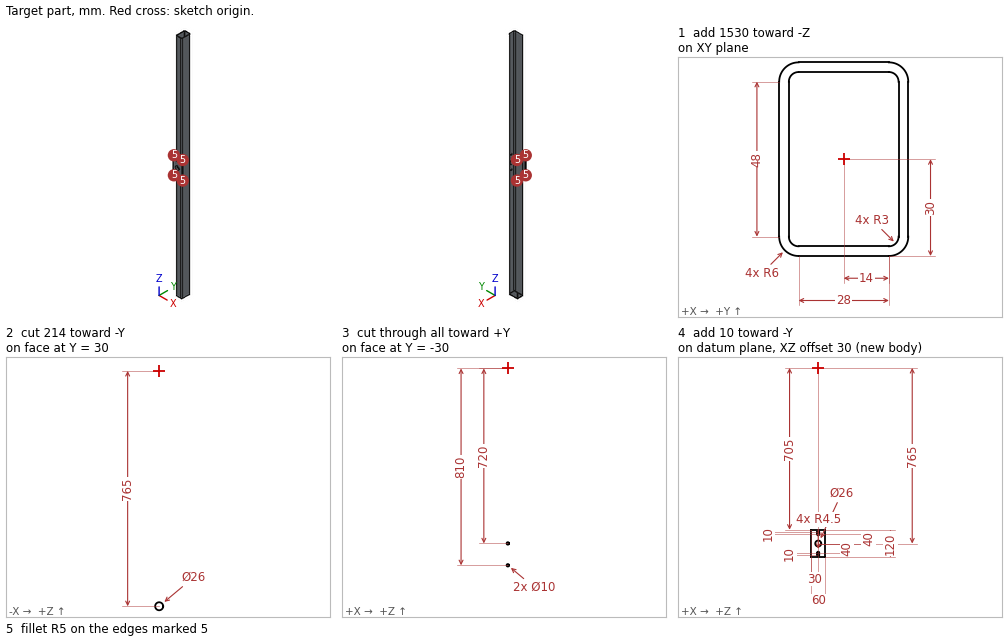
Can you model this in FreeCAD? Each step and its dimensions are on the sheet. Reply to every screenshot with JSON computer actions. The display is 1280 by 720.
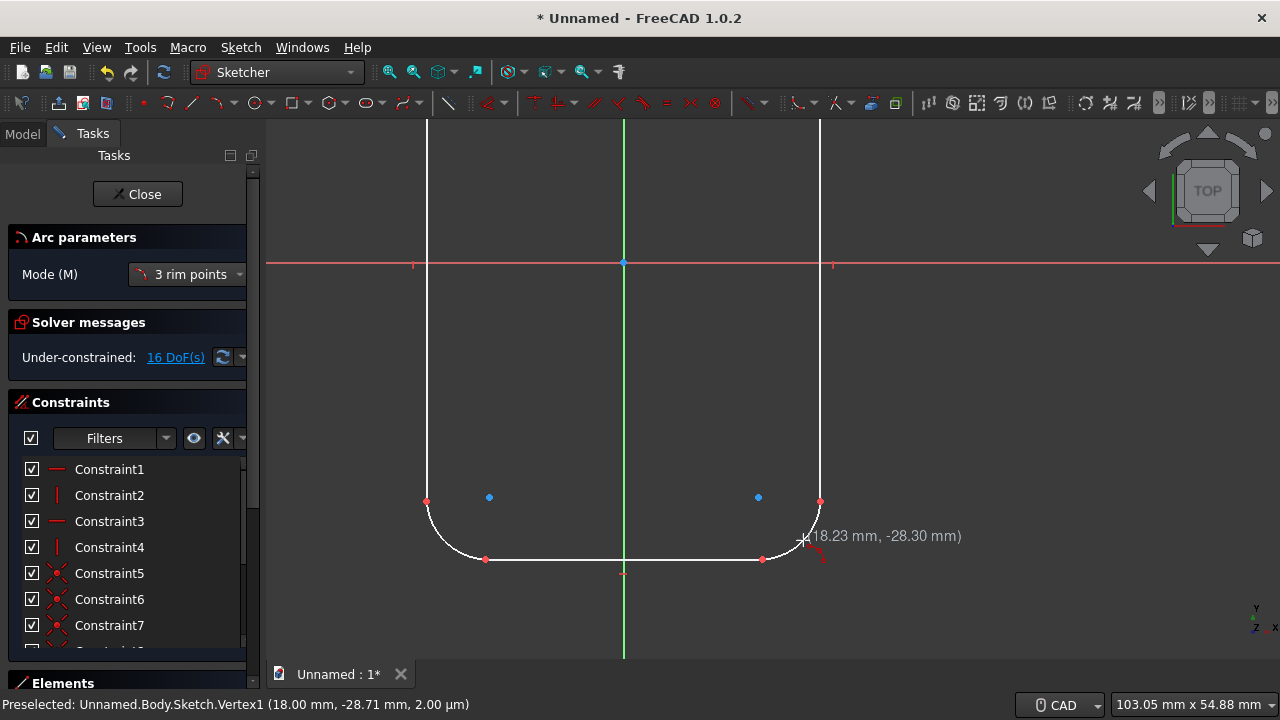
{"action": "left_click", "coordinate": [192, 104]}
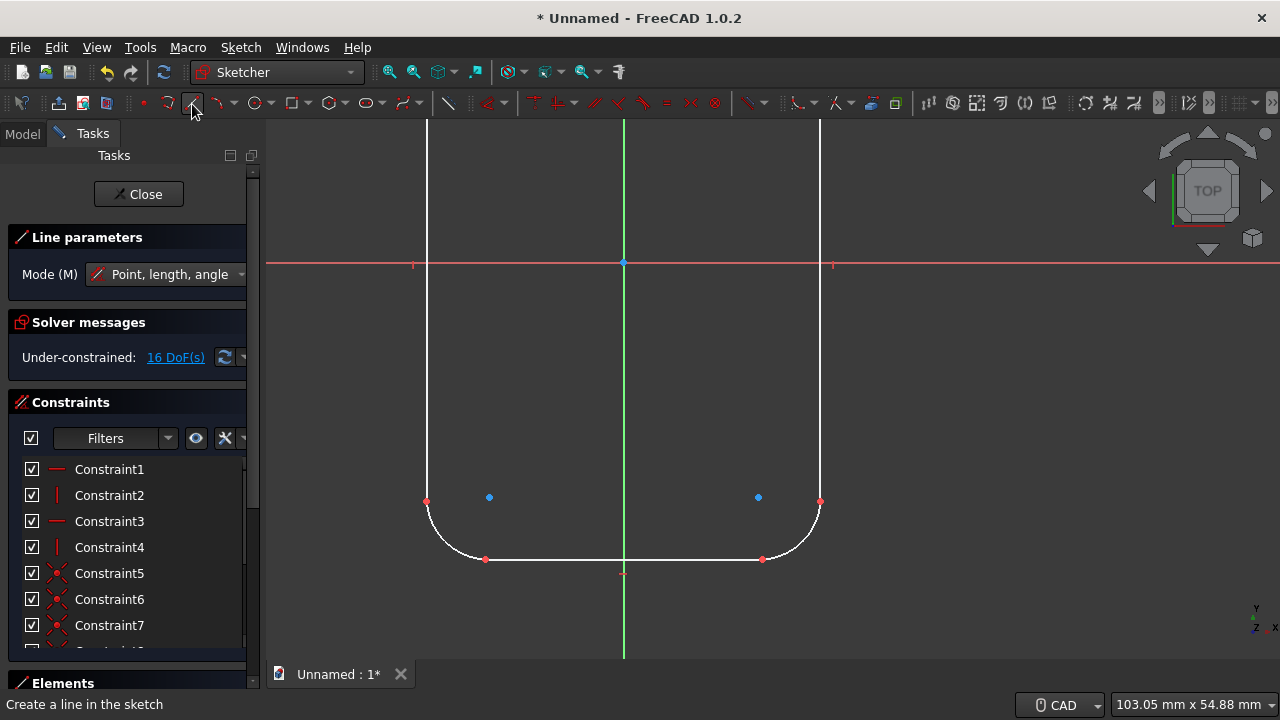
{"action": "left_click", "coordinate": [486, 528]}
{"action": "left_click", "coordinate": [761, 528]}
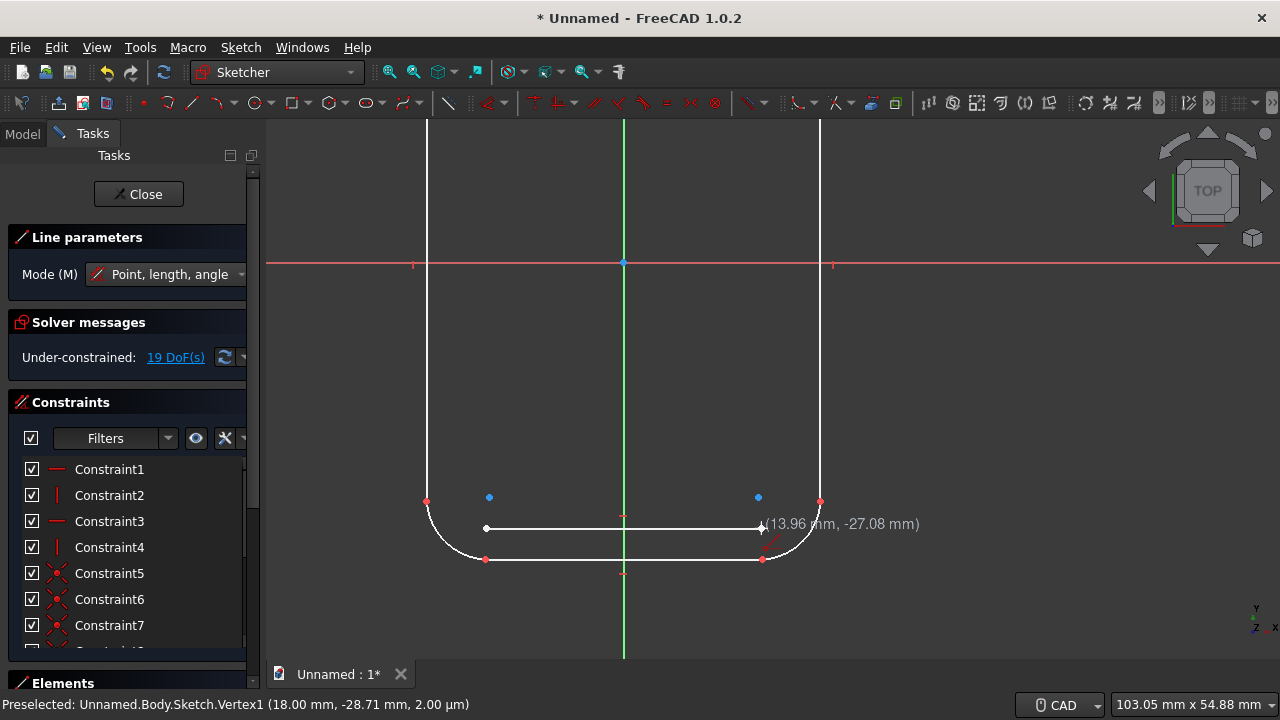
{"action": "left_click", "coordinate": [791, 499]}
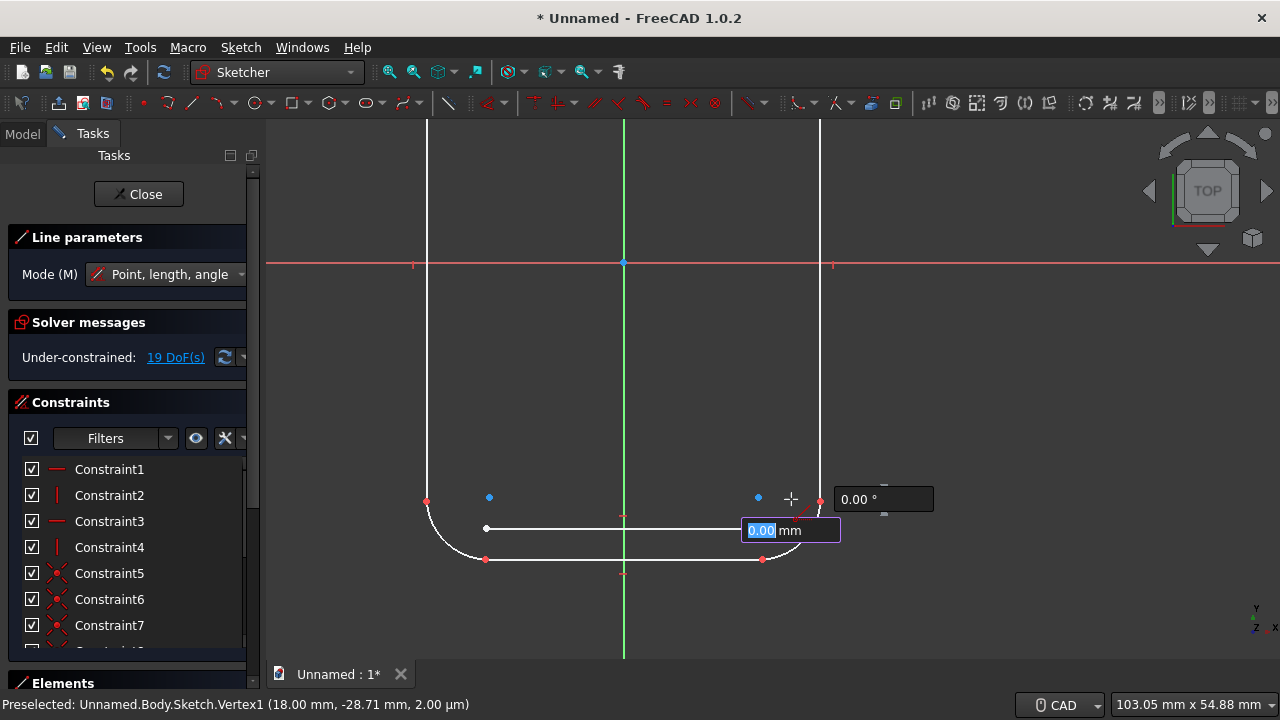
{"action": "scroll", "coordinate": [803, 543], "scroll_direction": "down", "scroll_amount": 3}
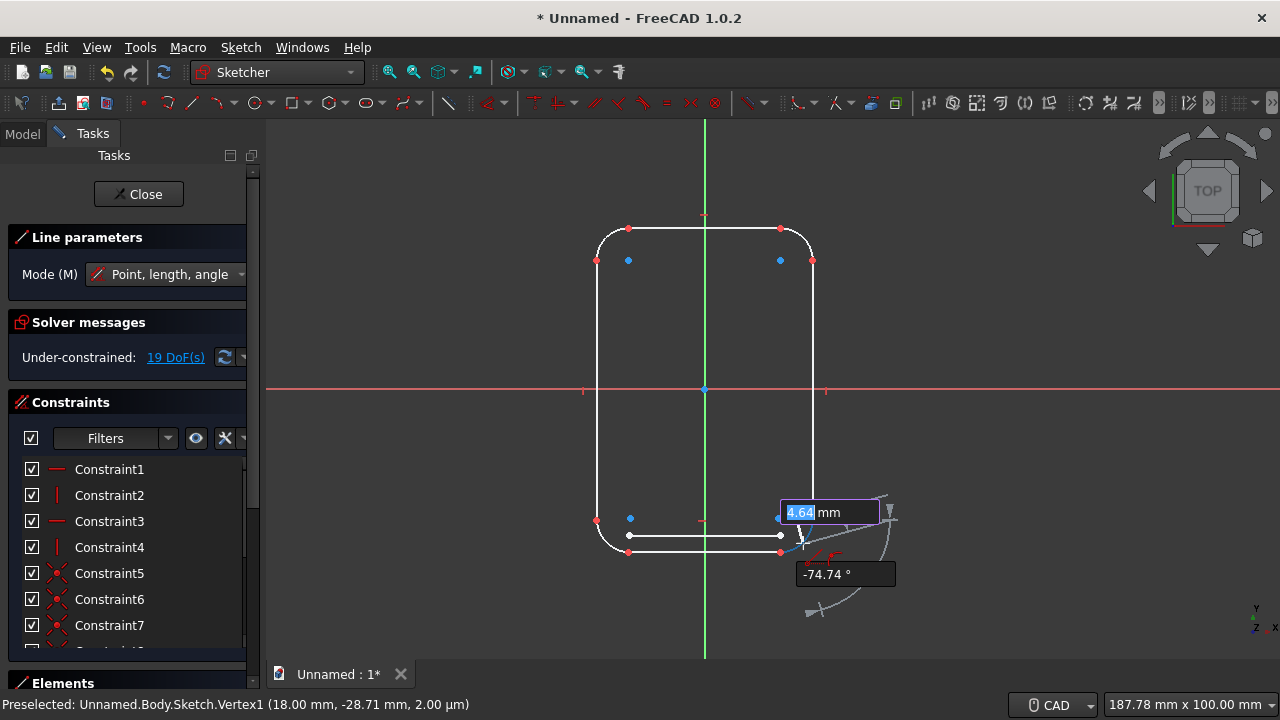
{"action": "left_click", "coordinate": [797, 260]}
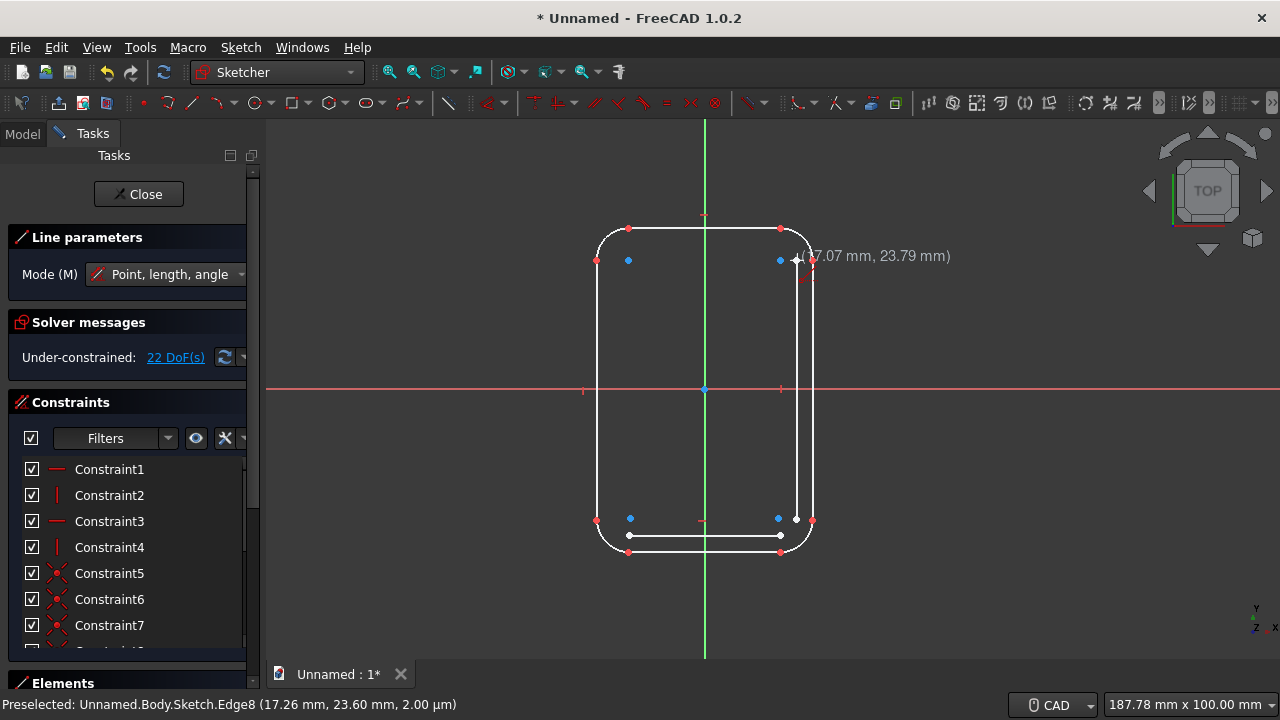
{"action": "left_click", "coordinate": [780, 244]}
{"action": "left_click", "coordinate": [629, 244]}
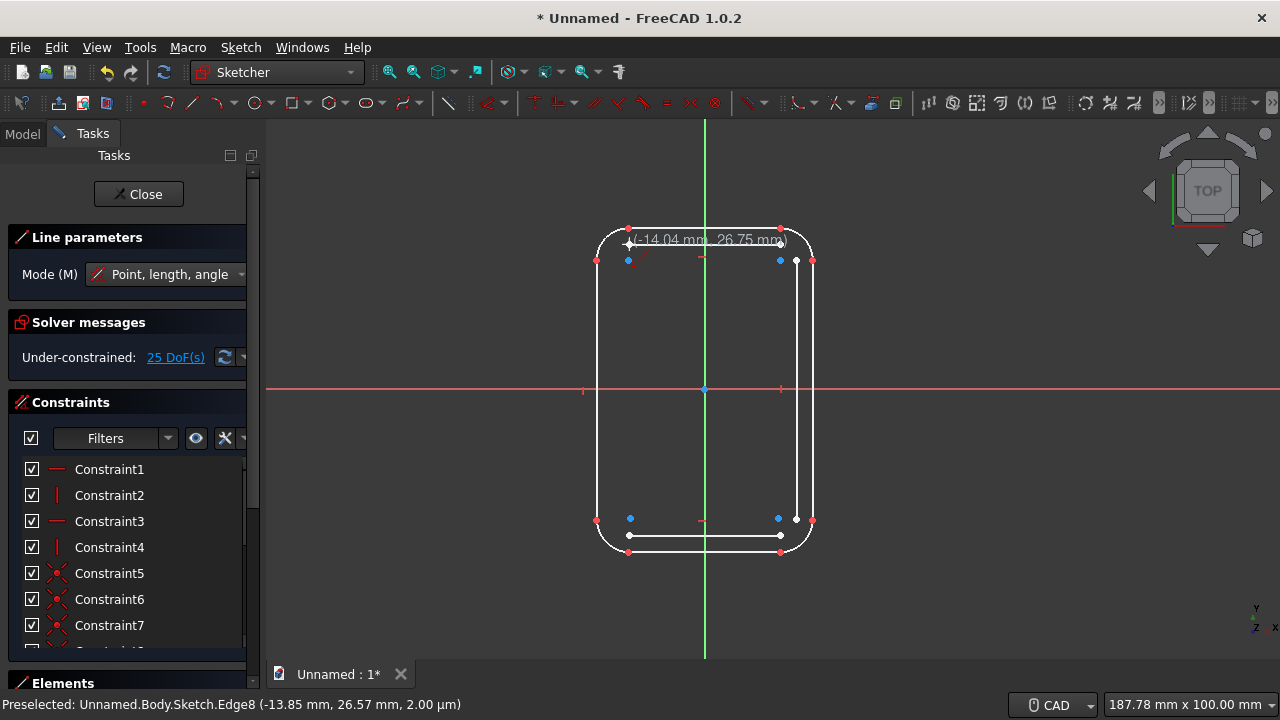
{"action": "left_click", "coordinate": [613, 260]}
{"action": "left_click", "coordinate": [613, 519]}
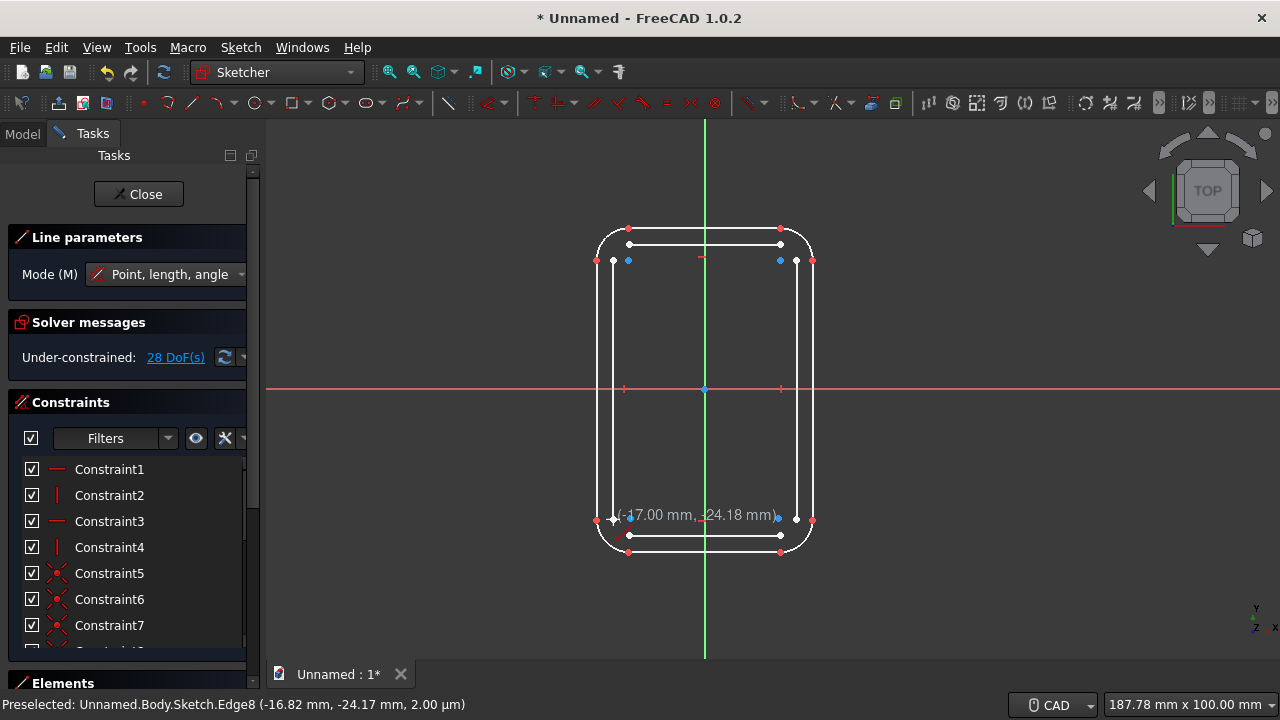
{"action": "left_click", "coordinate": [218, 104]}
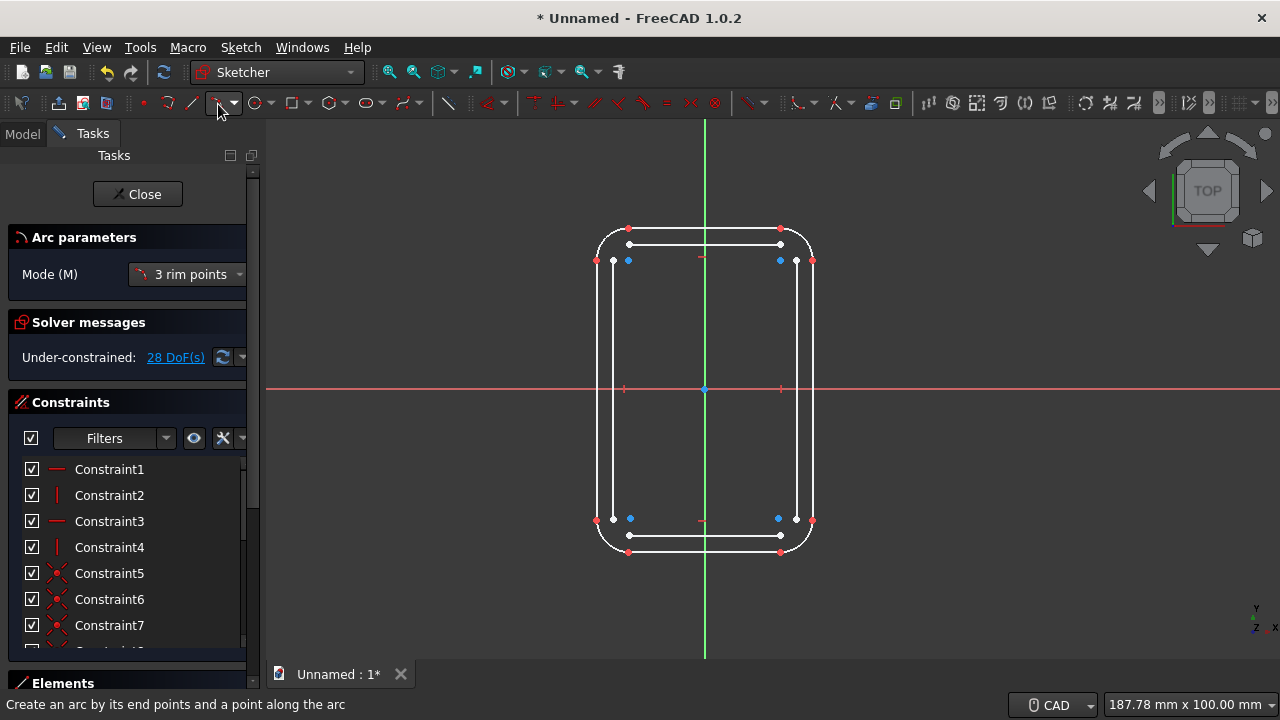
{"action": "left_click", "coordinate": [780, 536]}
{"action": "left_click", "coordinate": [797, 520]}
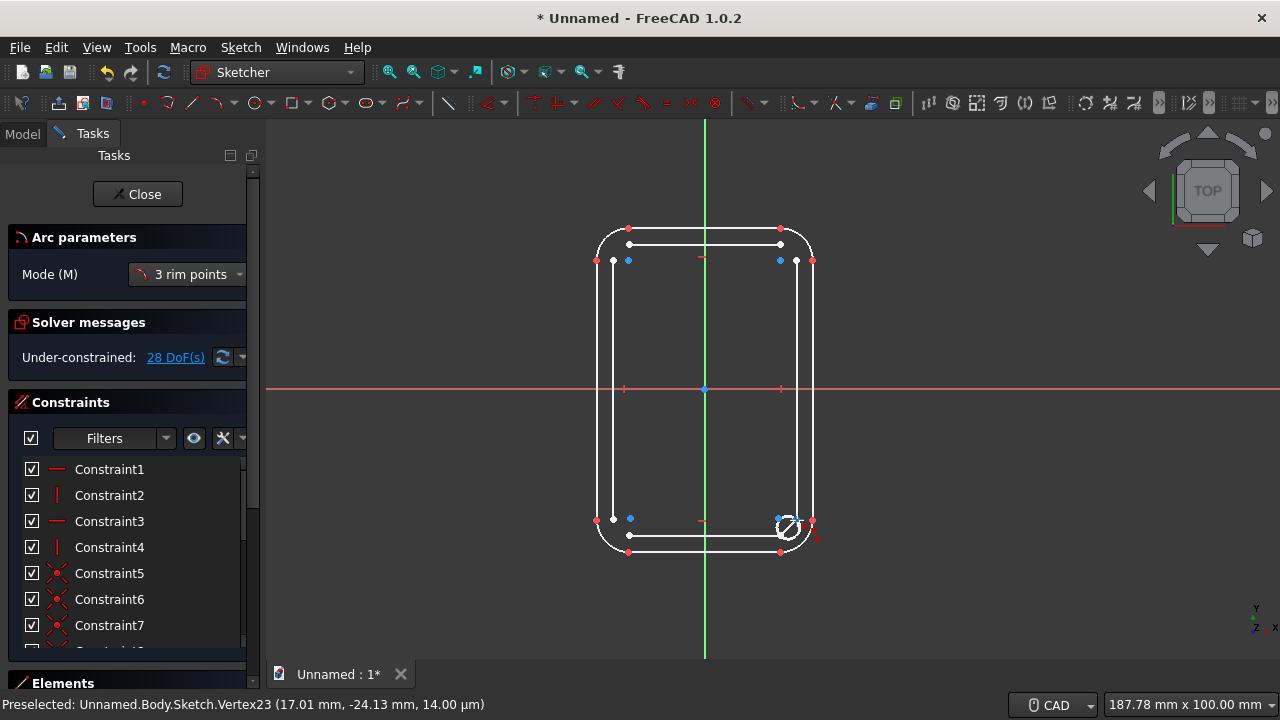
{"action": "scroll", "coordinate": [792, 531], "scroll_direction": "up", "scroll_amount": 7}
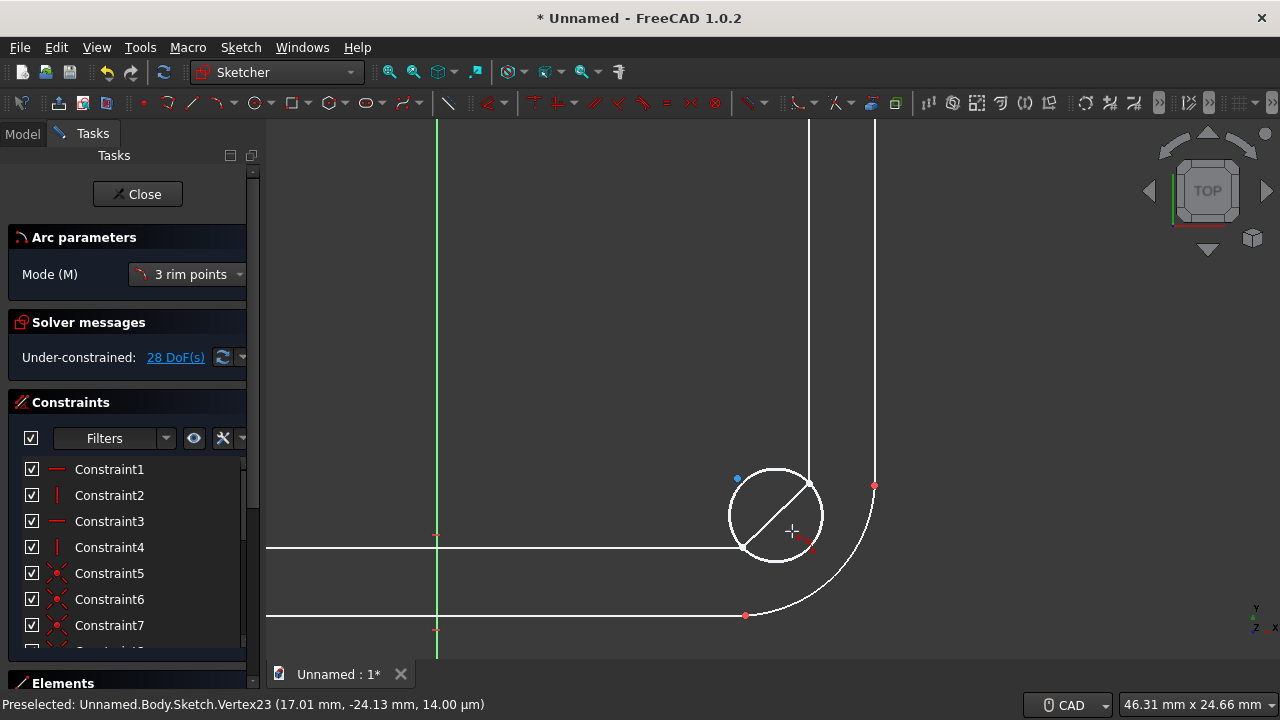
{"action": "left_click", "coordinate": [790, 527]}